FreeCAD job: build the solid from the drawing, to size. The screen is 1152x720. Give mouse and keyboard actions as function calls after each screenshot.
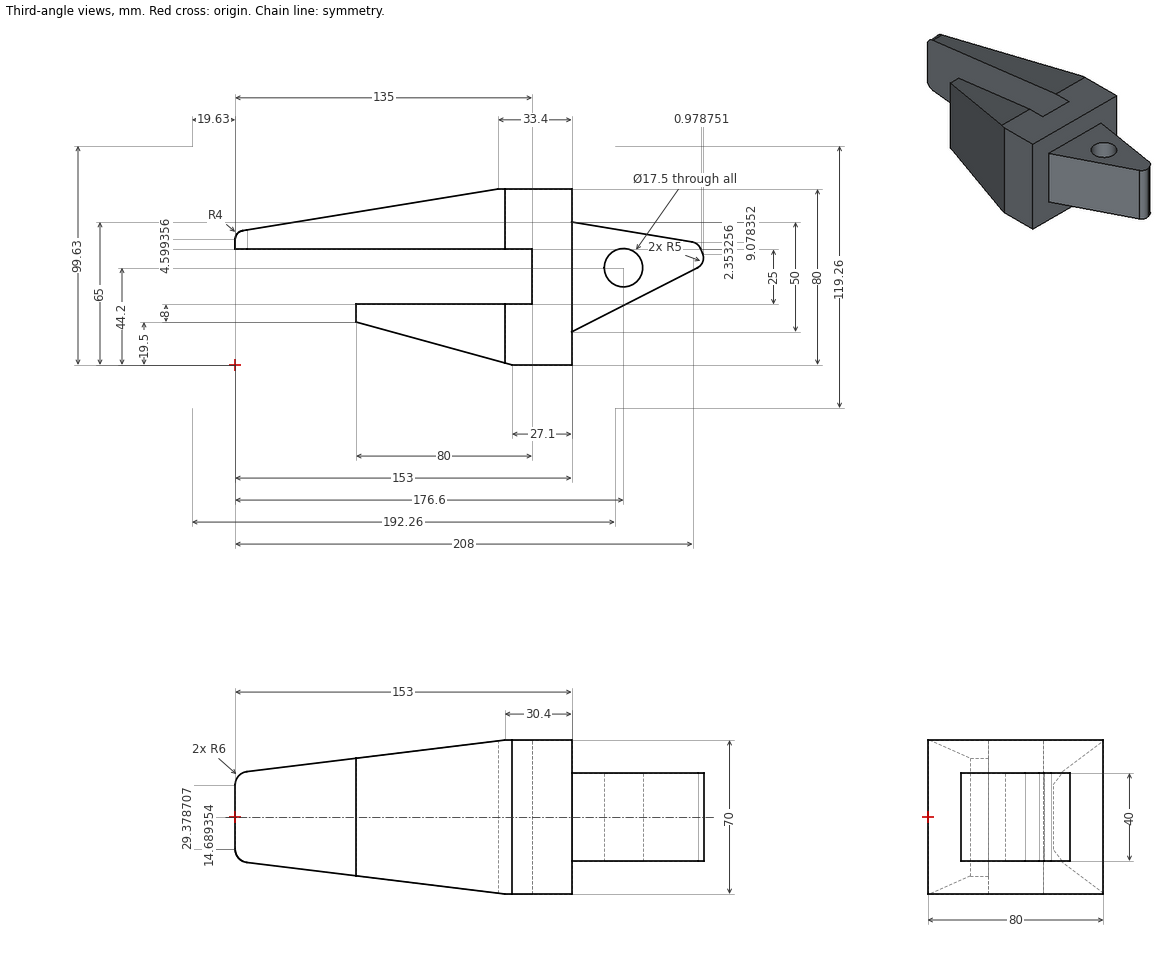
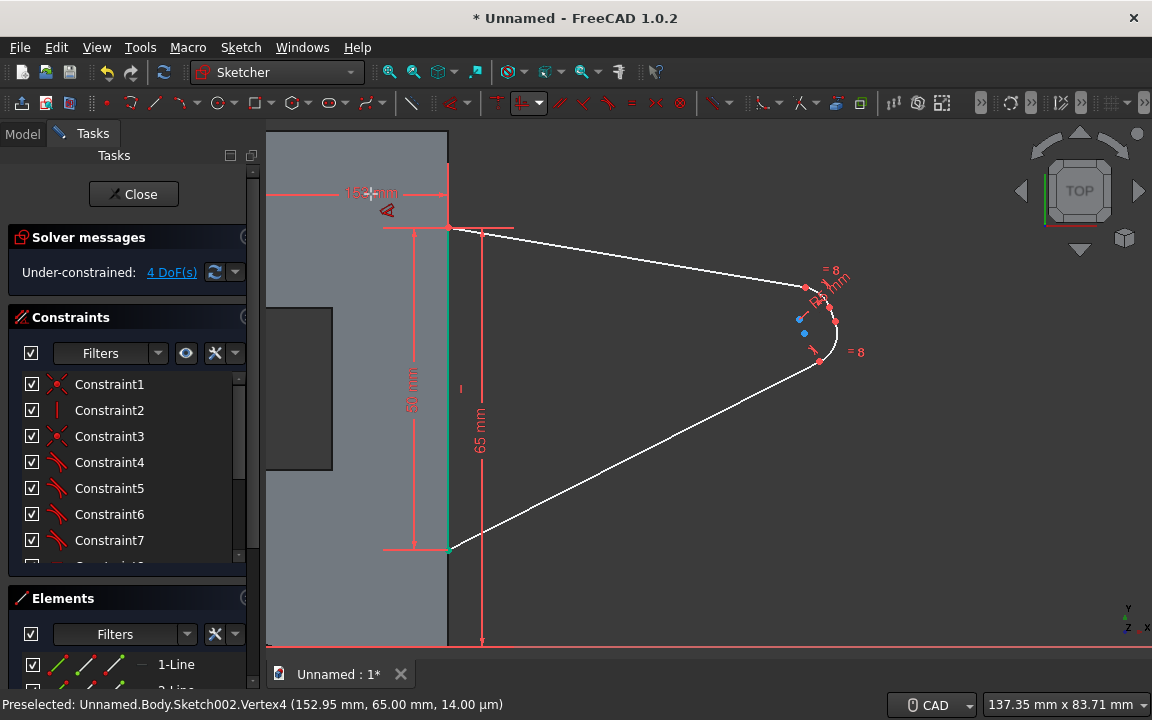
click(805, 333)
click(549, 299)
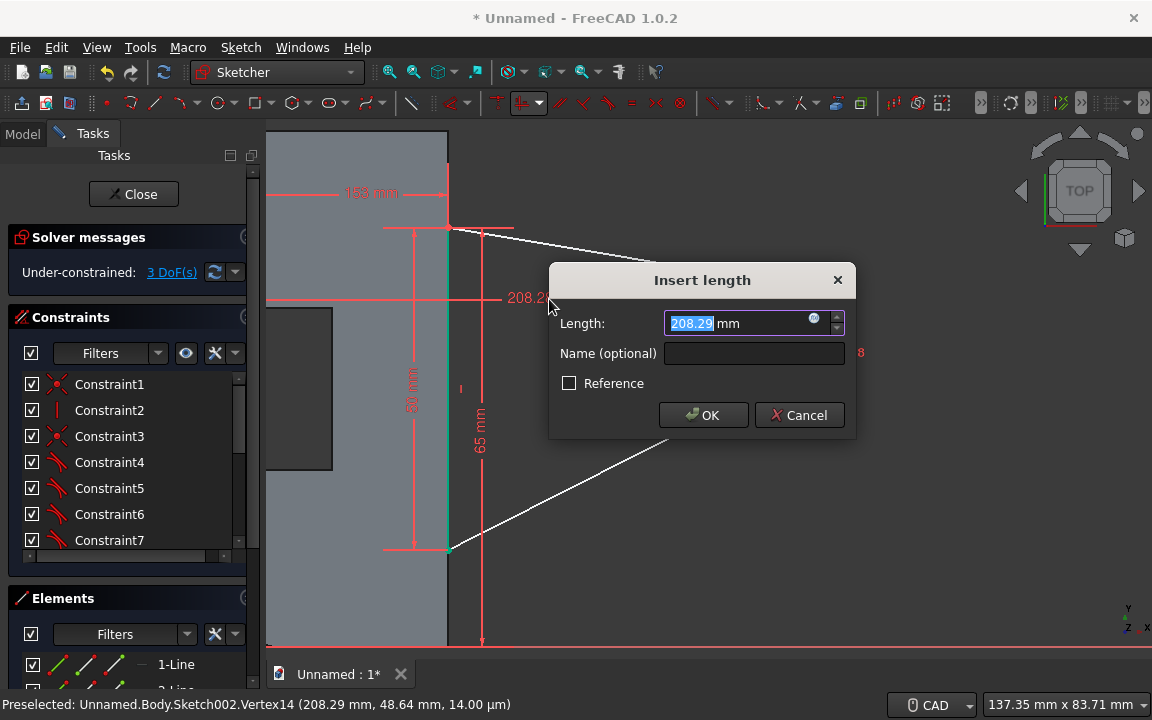
text(208)
key(Return)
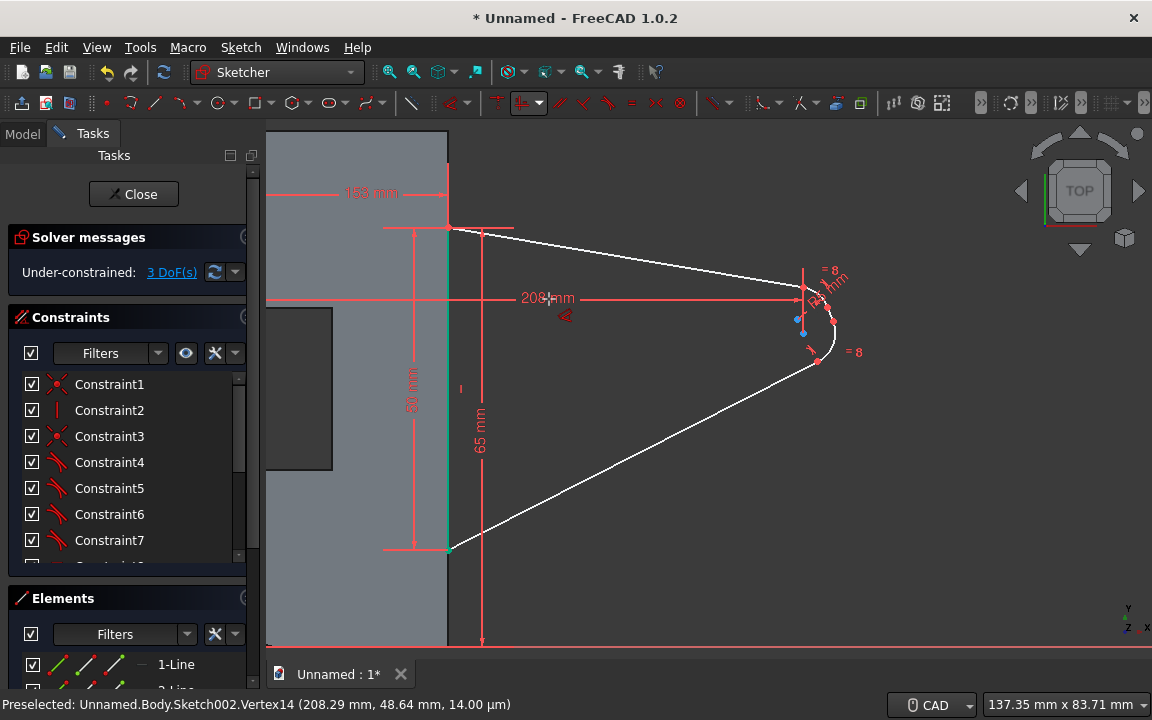
scroll(831, 315, up, 10)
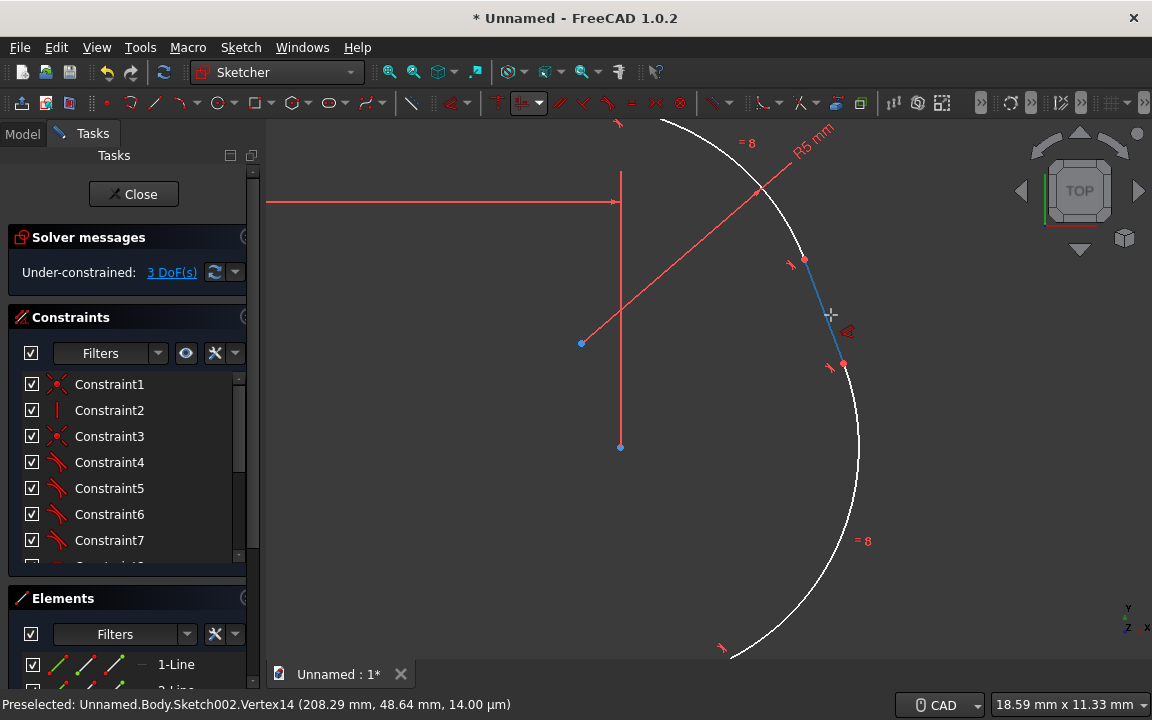
click(824, 311)
click(824, 226)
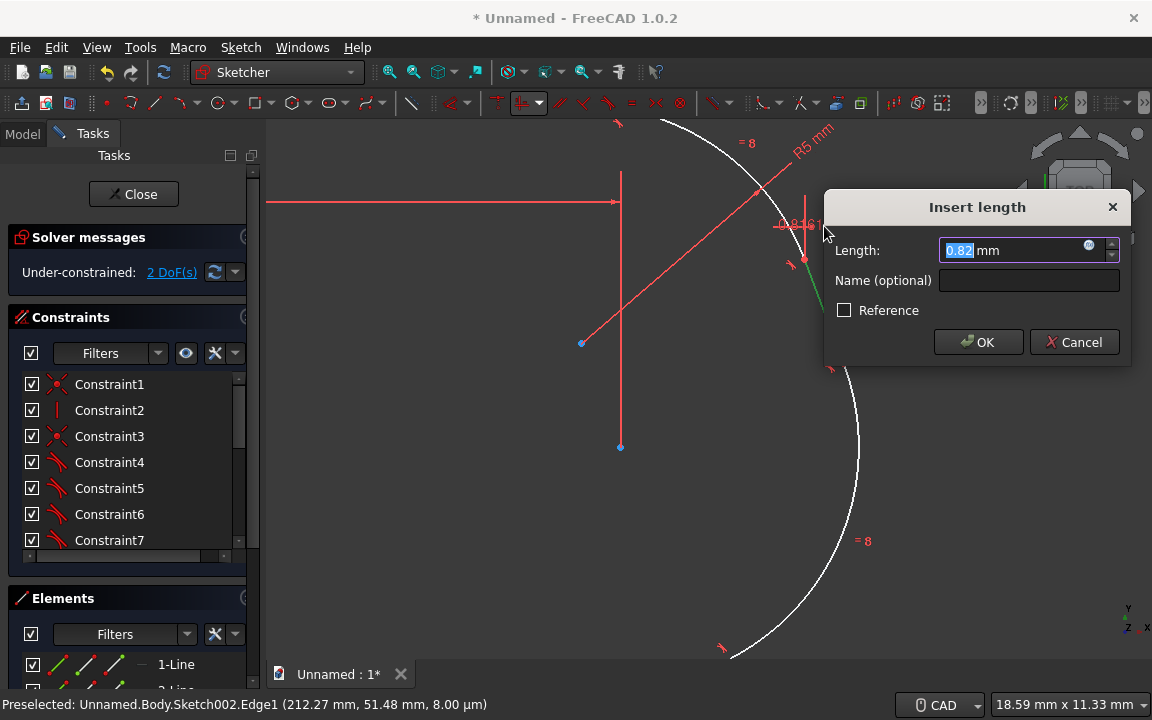
text(0.978751)
key(Return)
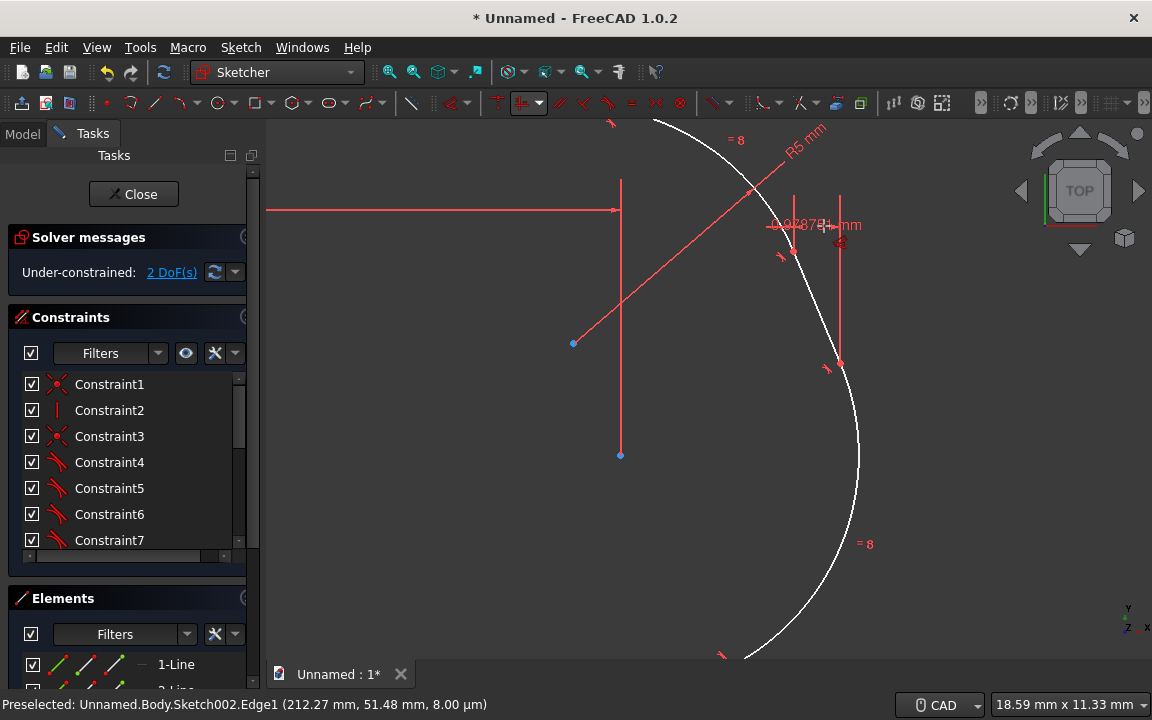
click(826, 330)
click(874, 307)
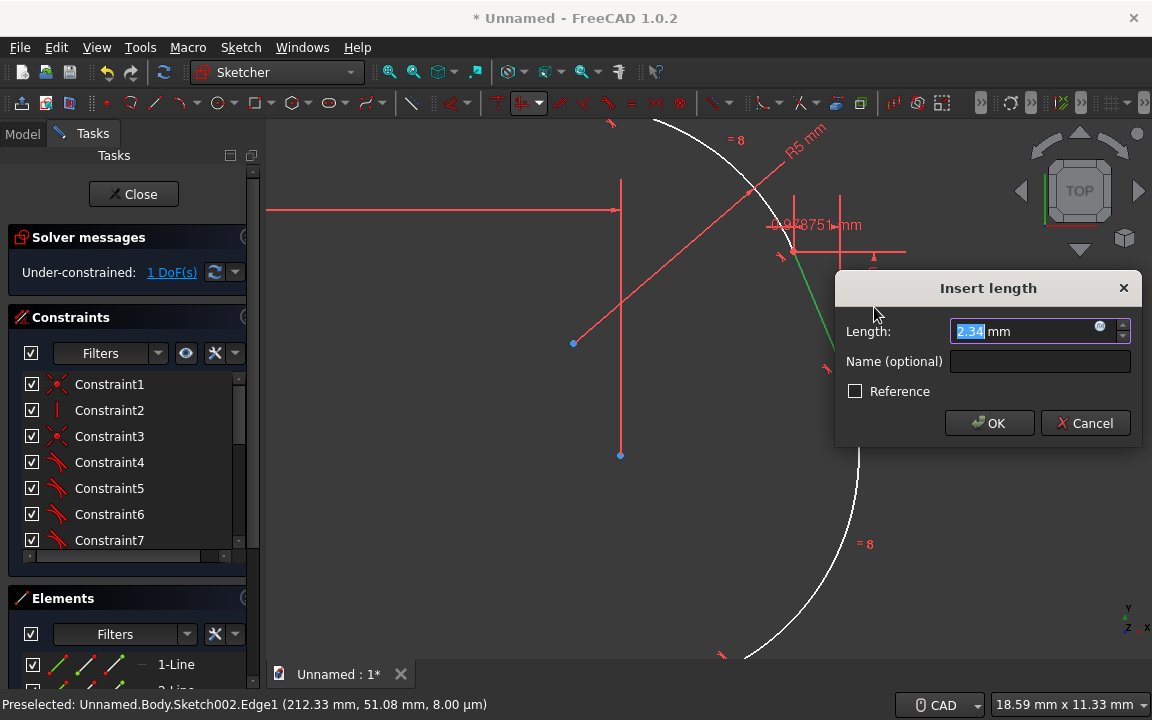
text(2.353256)
key(Return)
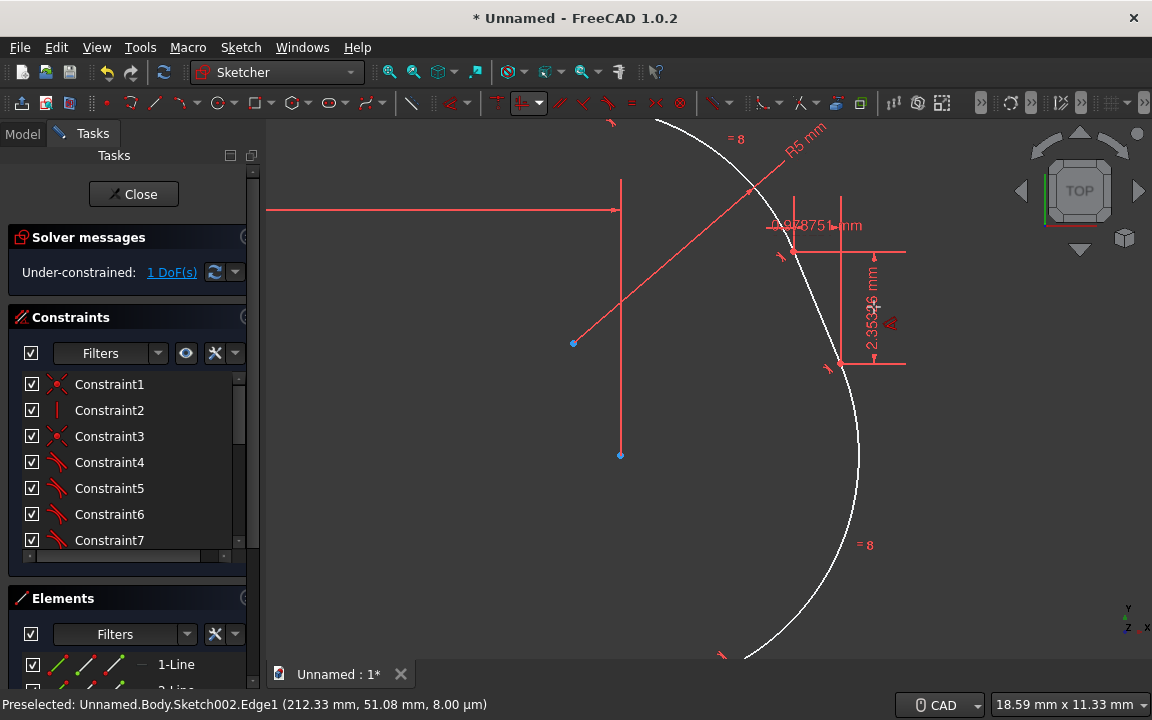
scroll(831, 315, down, 10)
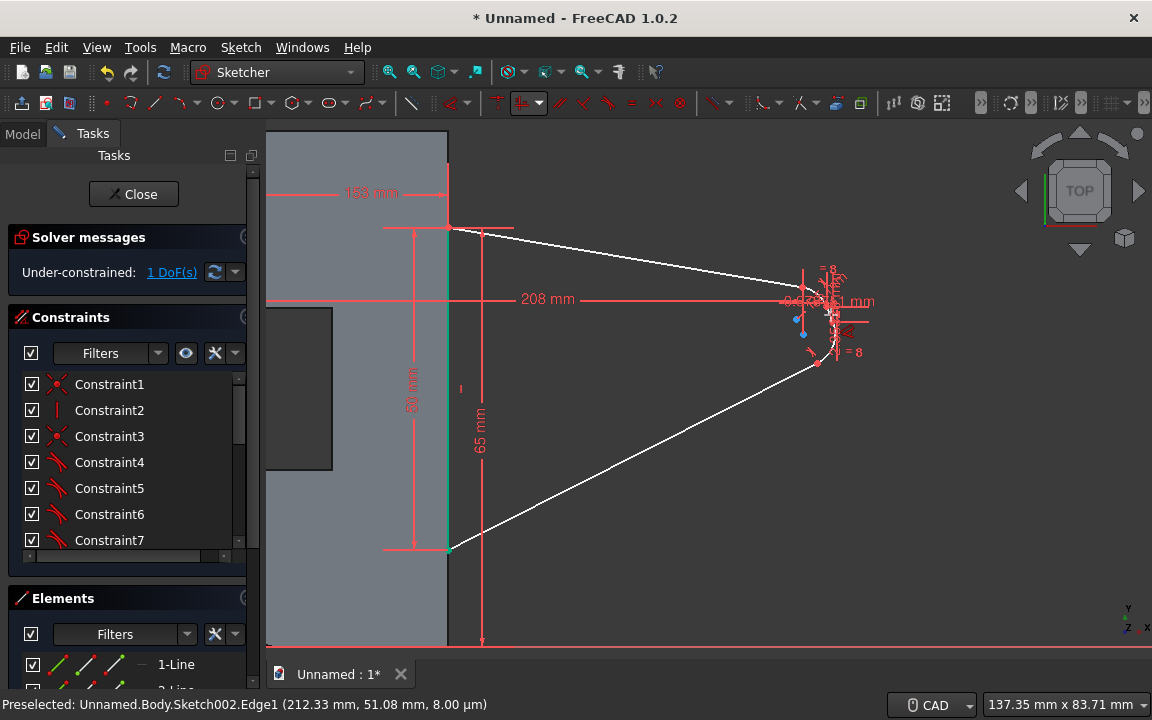
click(696, 269)
click(414, 257)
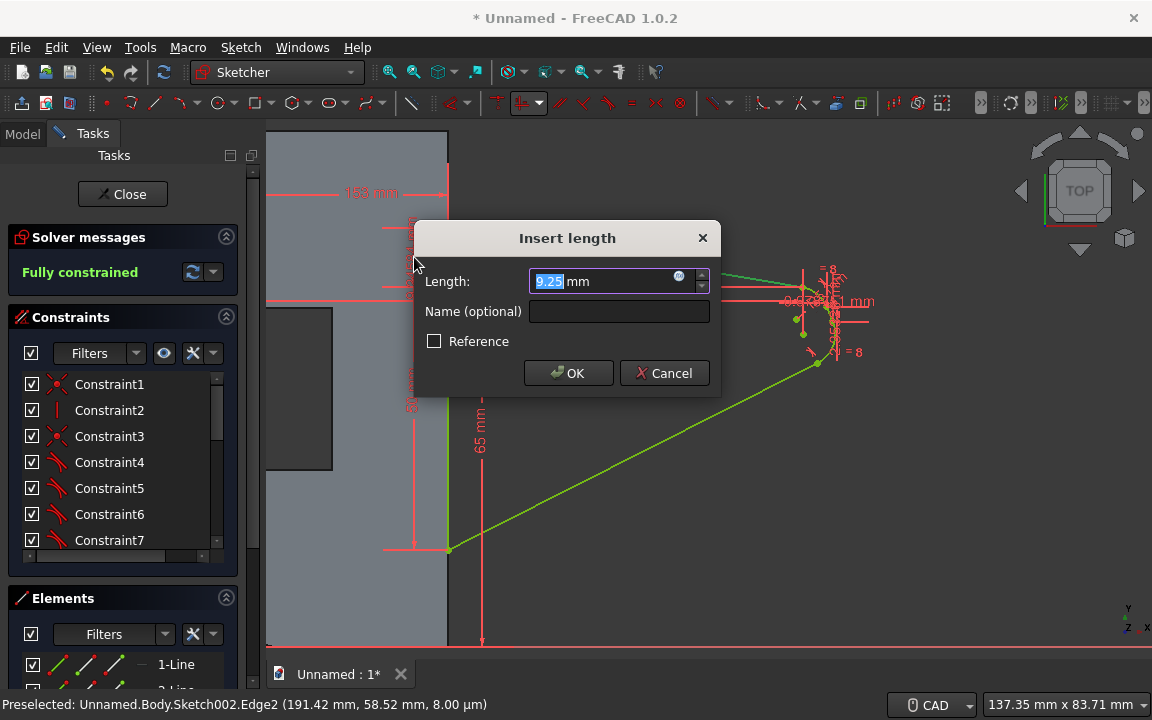
text(9.078352)
key(Return)
key(Escape)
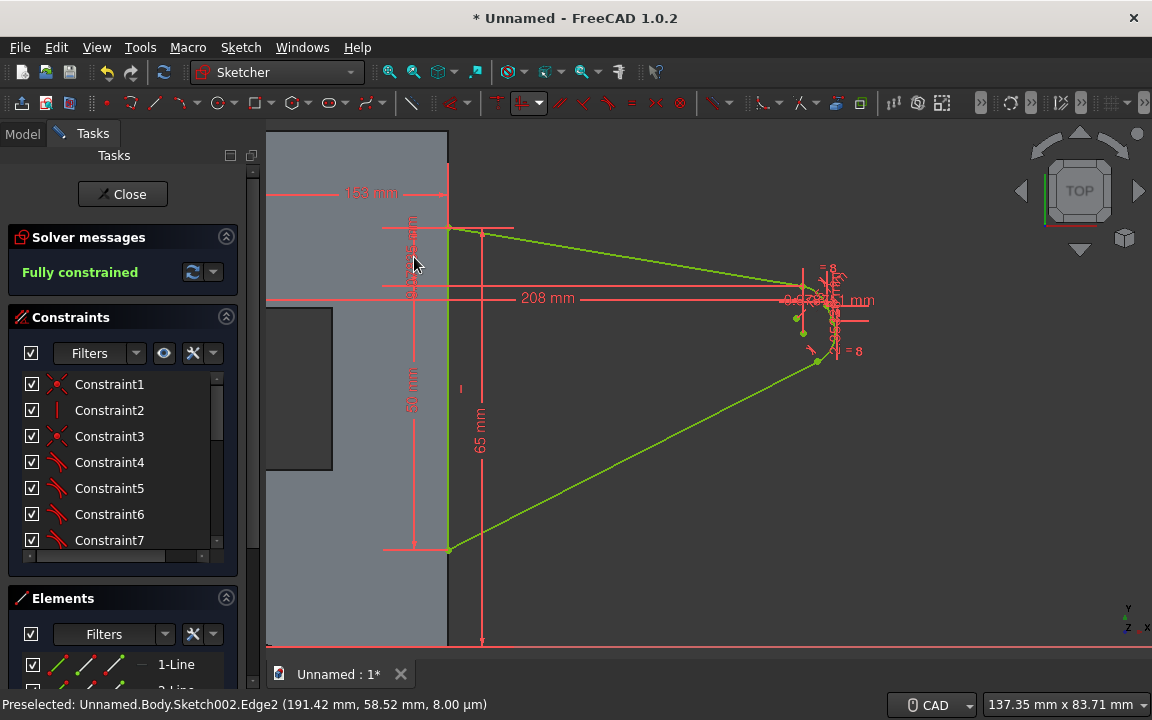
click(123, 194)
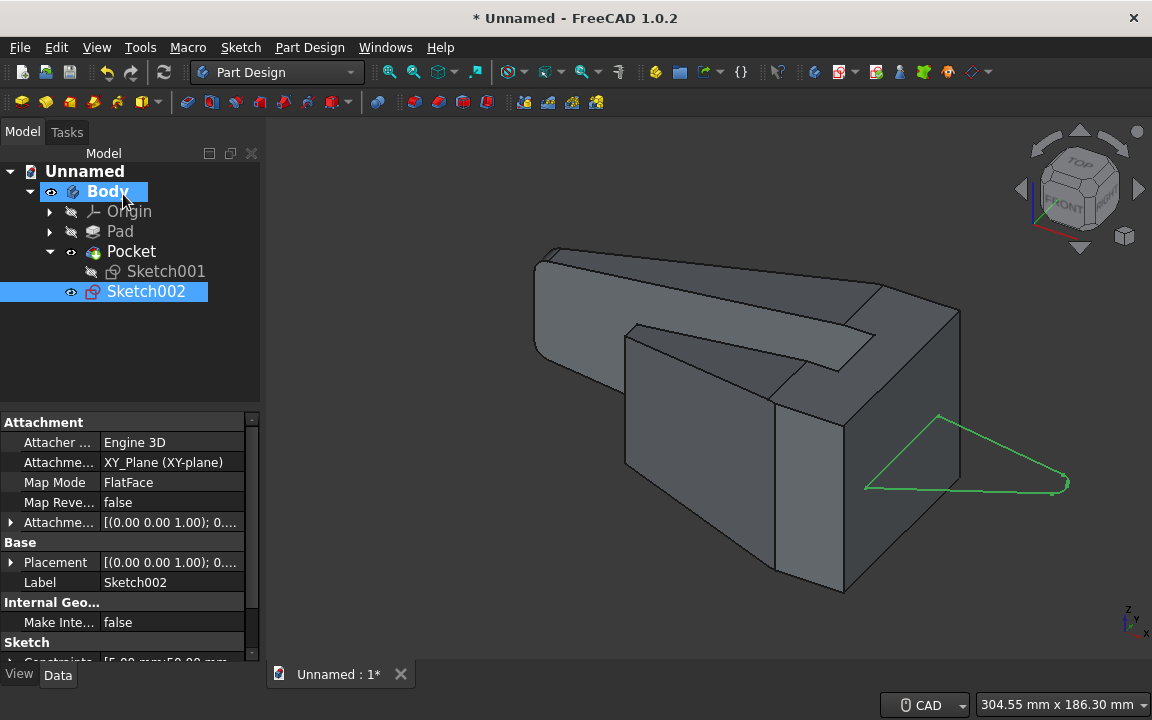
click(22, 102)